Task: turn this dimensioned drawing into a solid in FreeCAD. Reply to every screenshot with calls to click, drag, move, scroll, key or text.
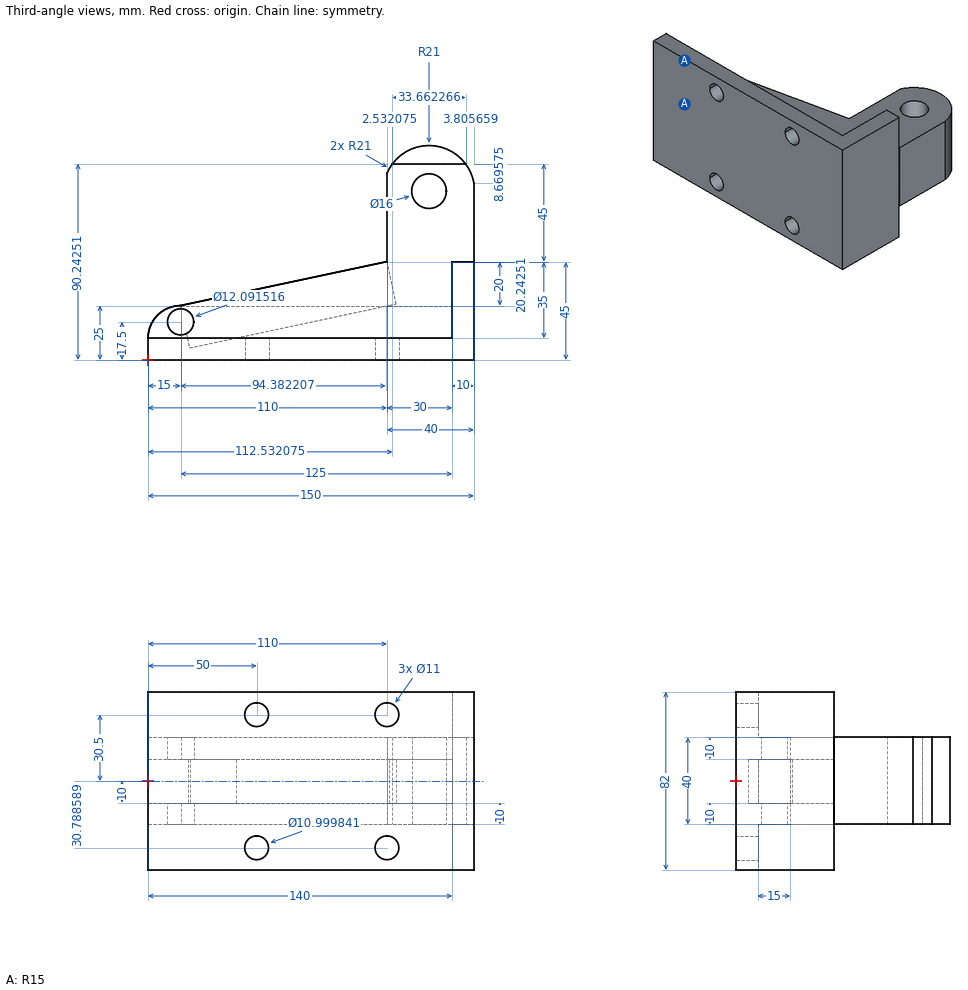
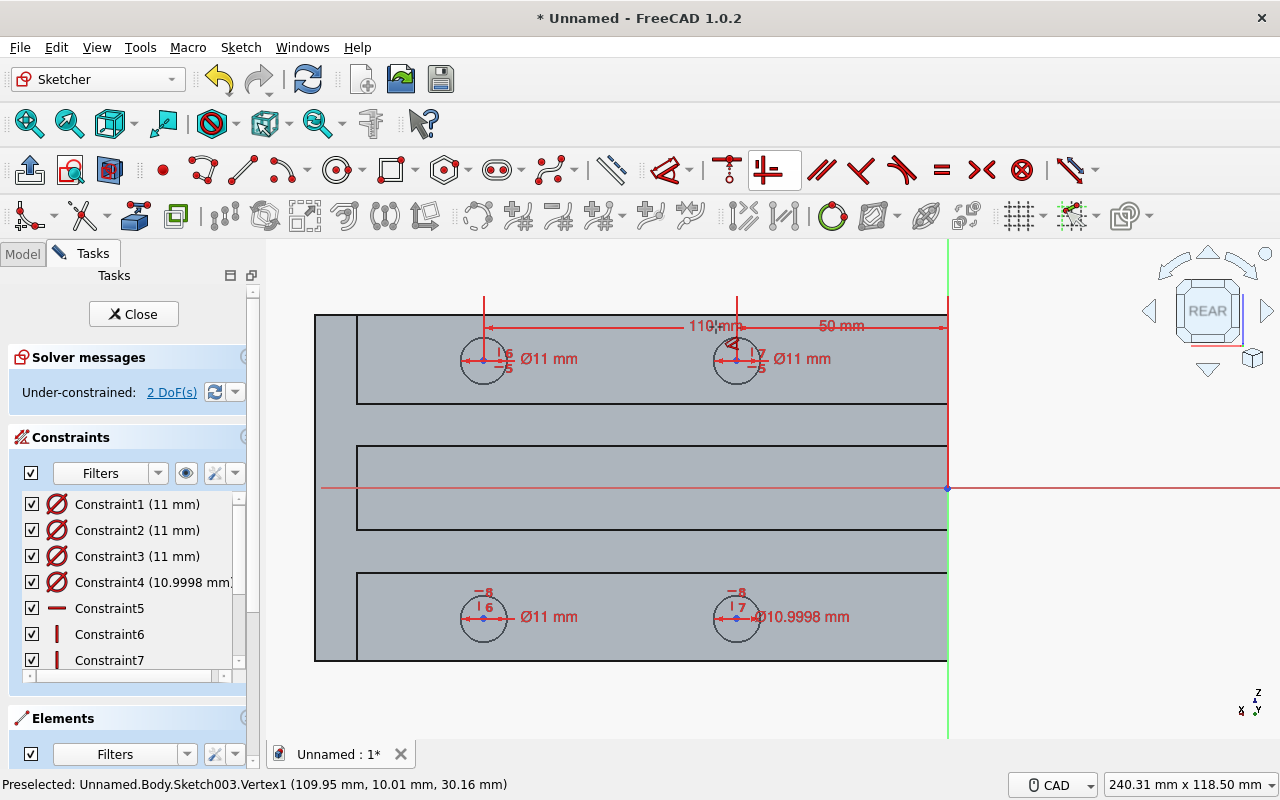
click(484, 361)
click(982, 425)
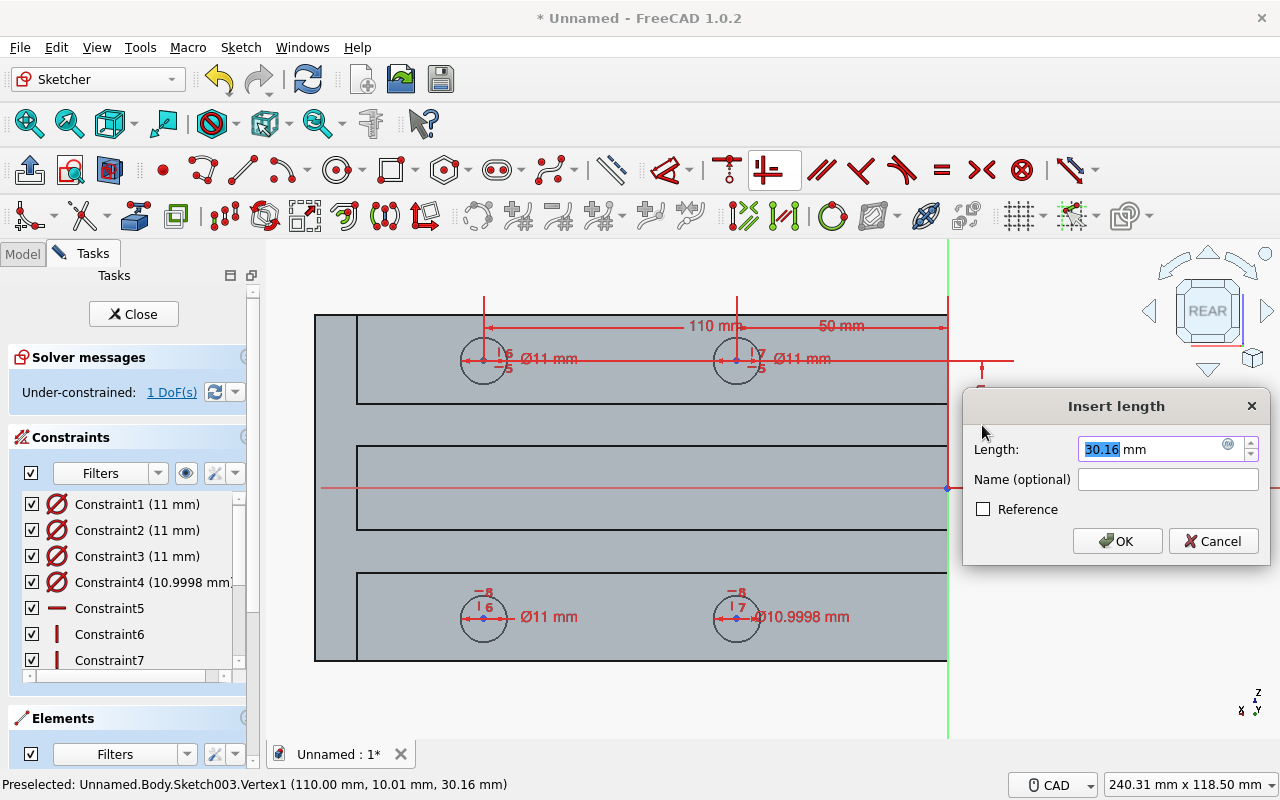
text(30.5)
key(Return)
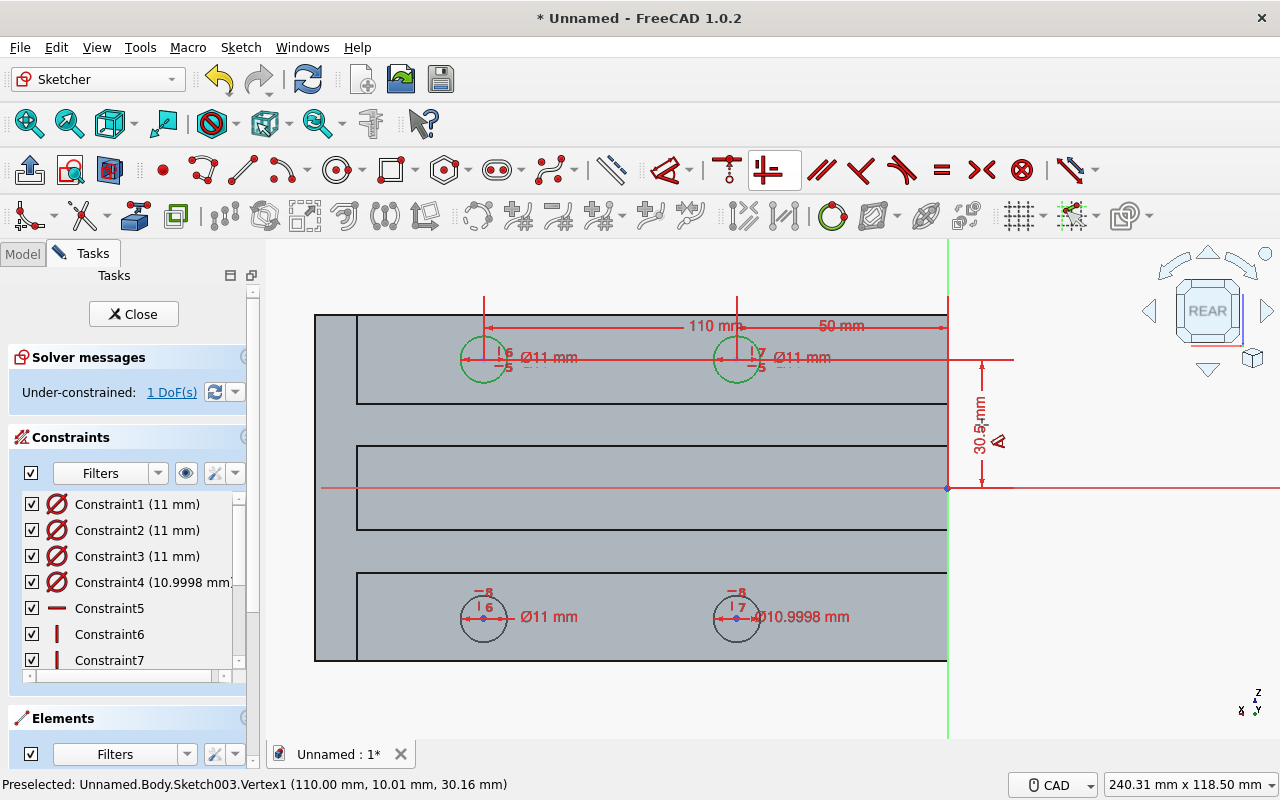
click(484, 619)
click(982, 554)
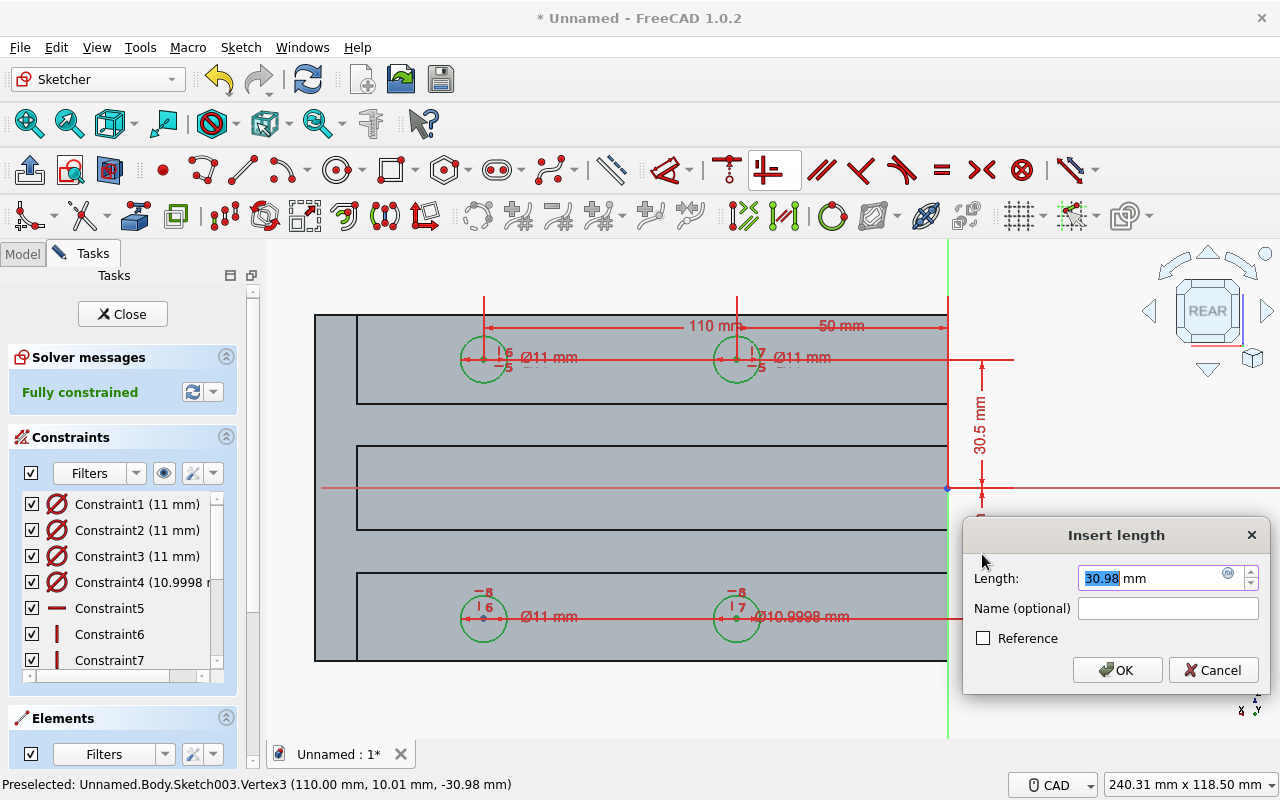
text(30.788589)
key(Return)
key(Escape)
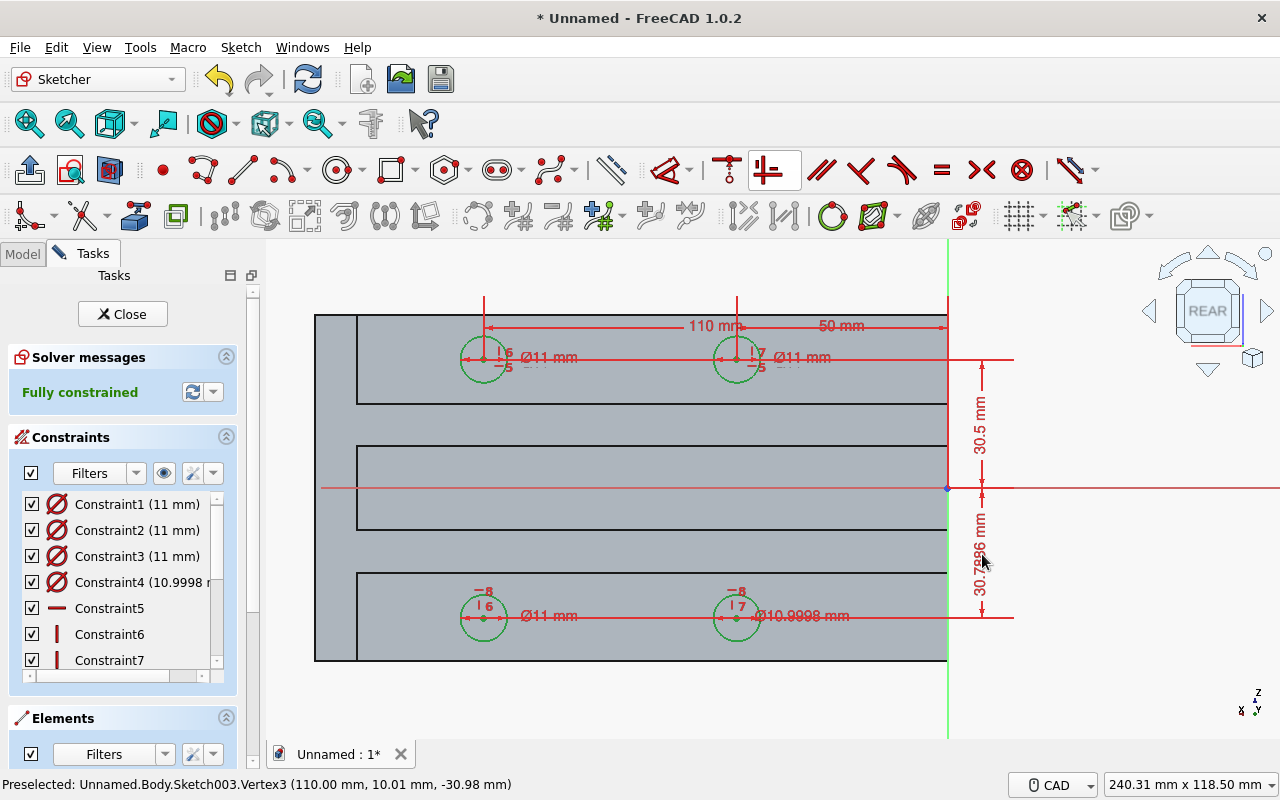
click(123, 314)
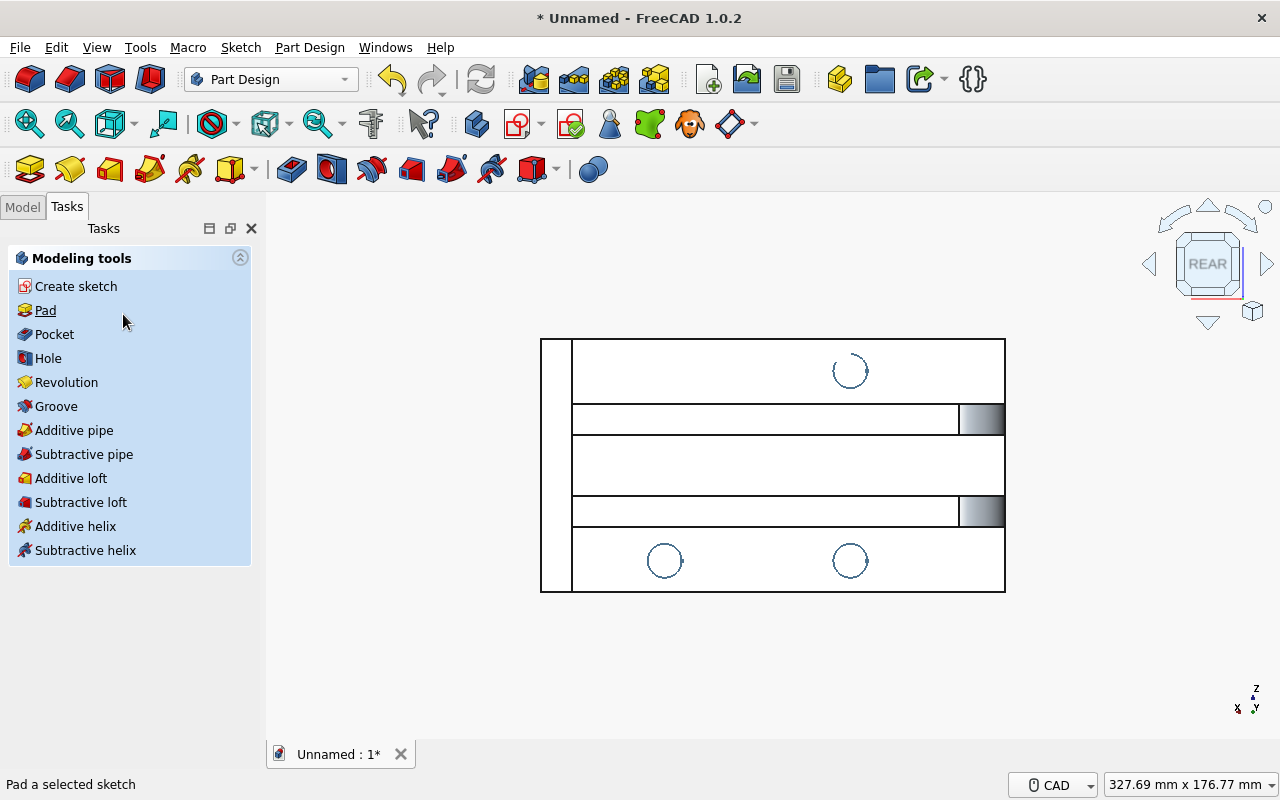
click(292, 170)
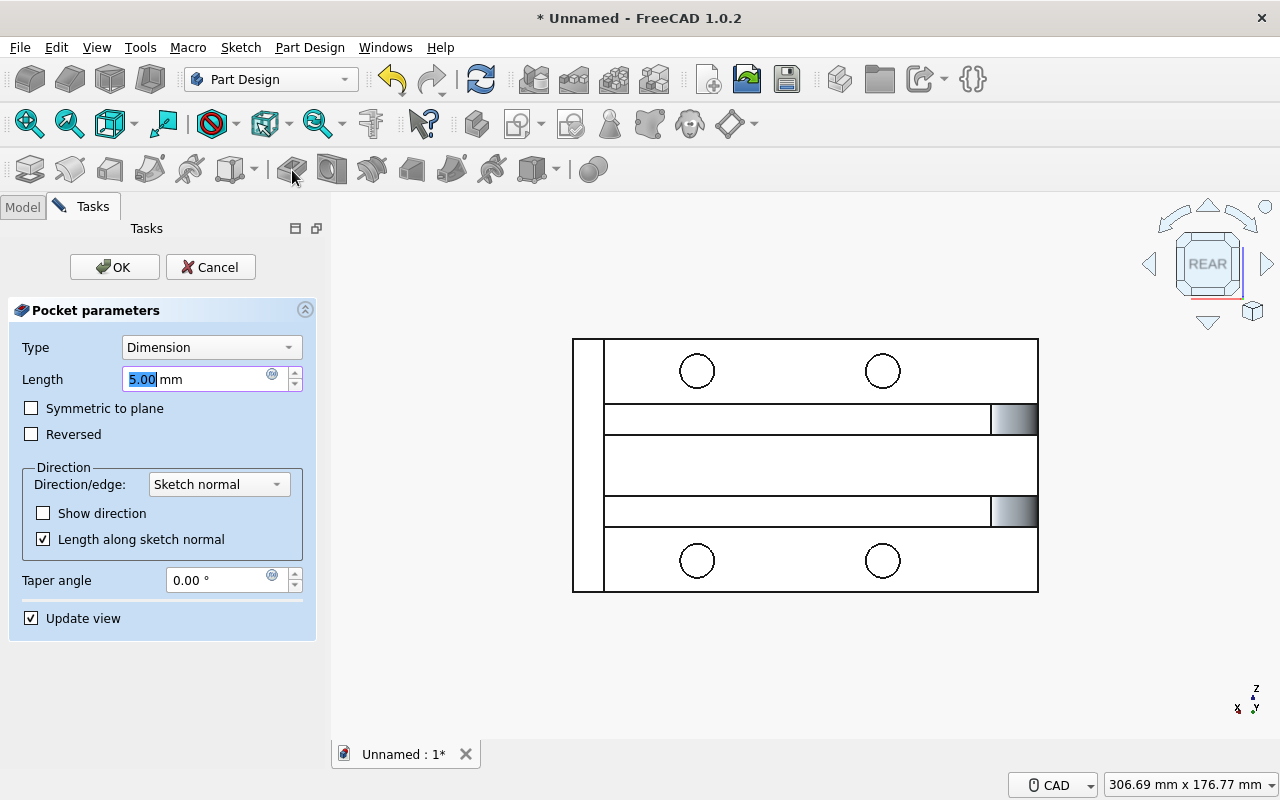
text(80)
key(Tab)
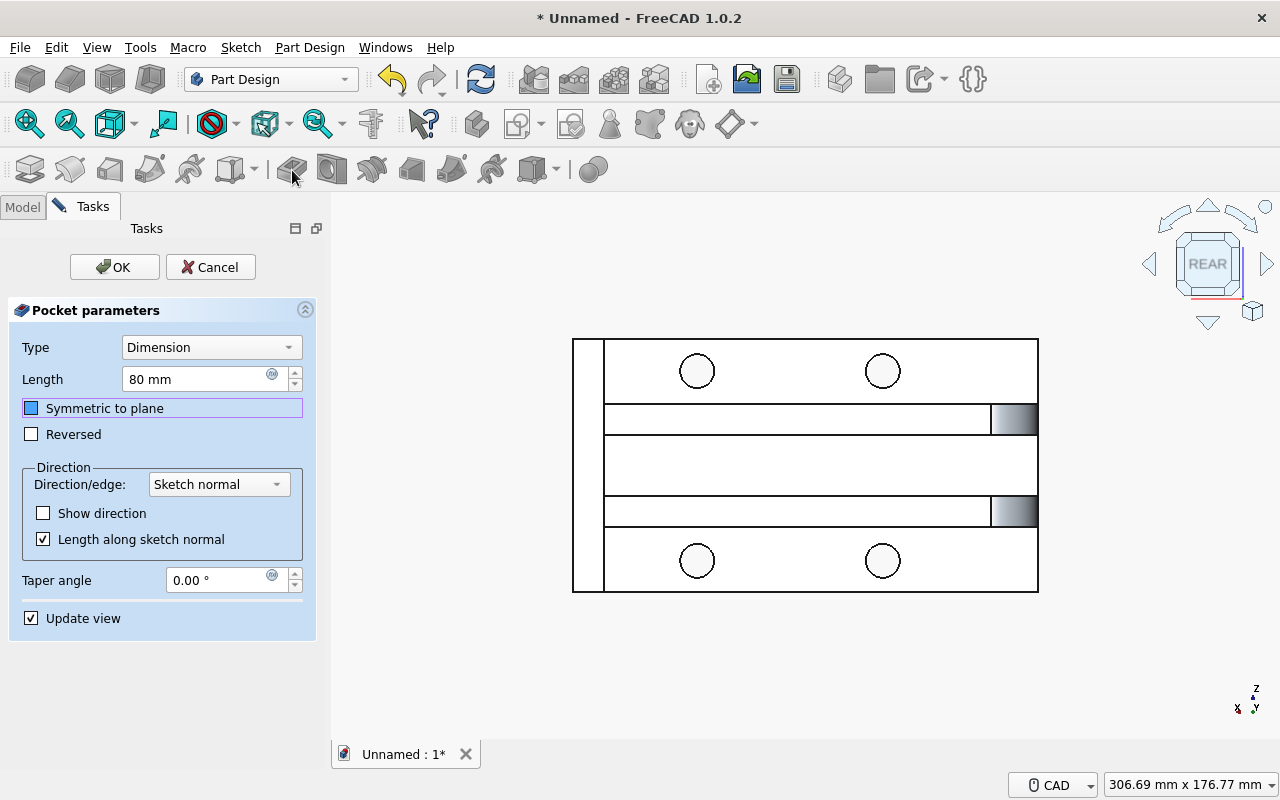
click(115, 267)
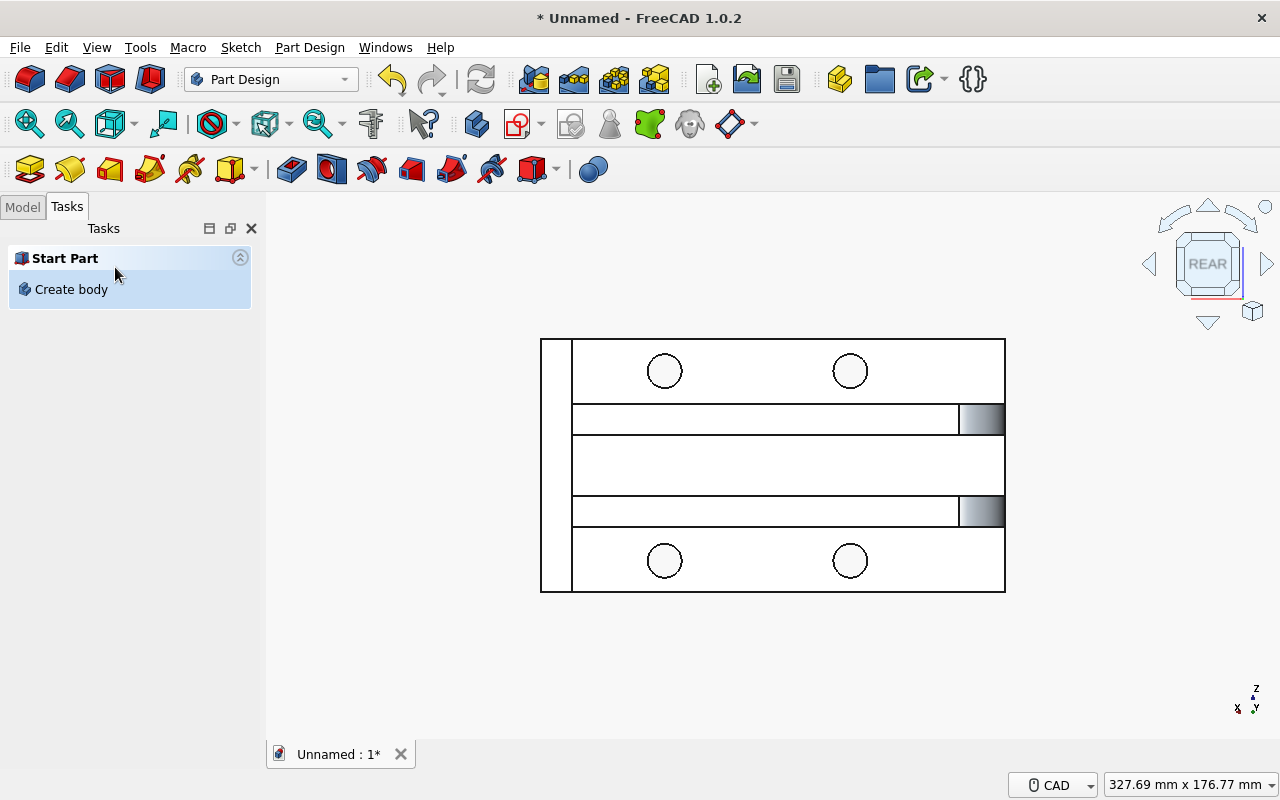
key(0)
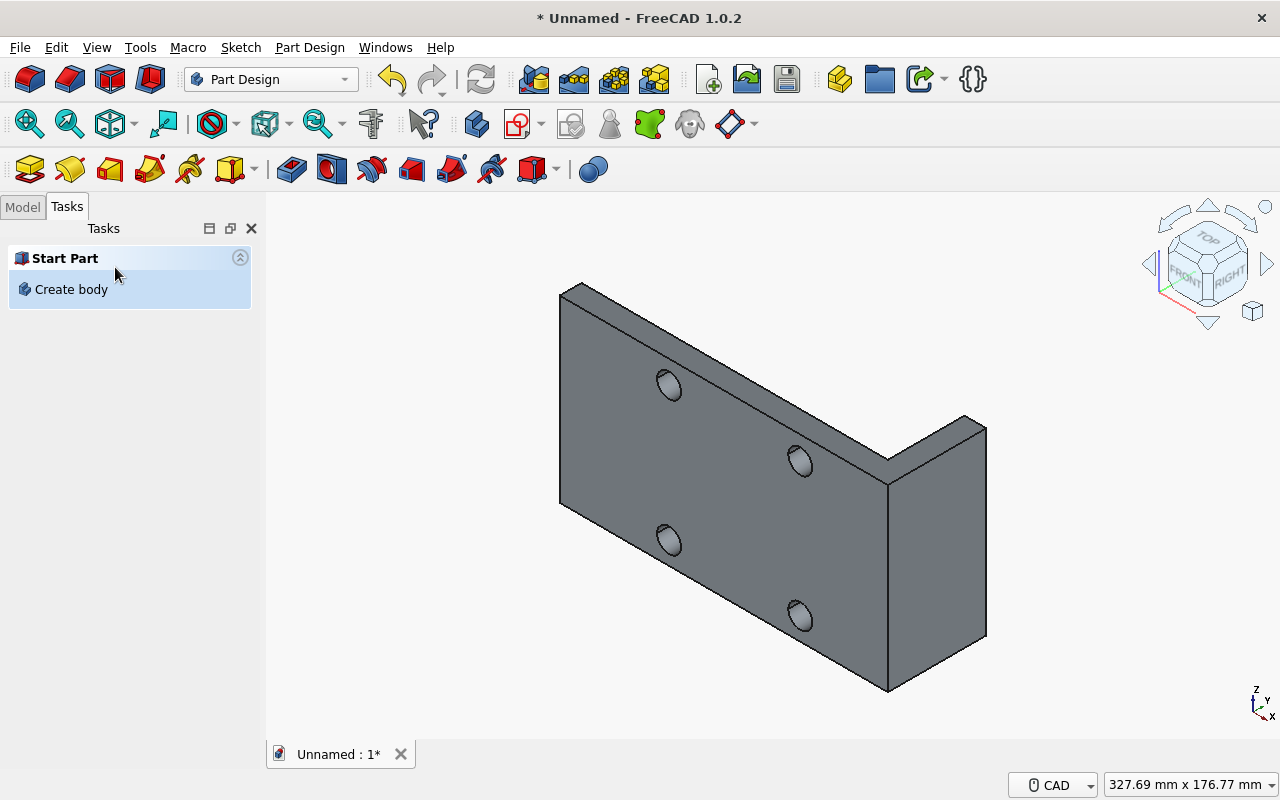
key(2)